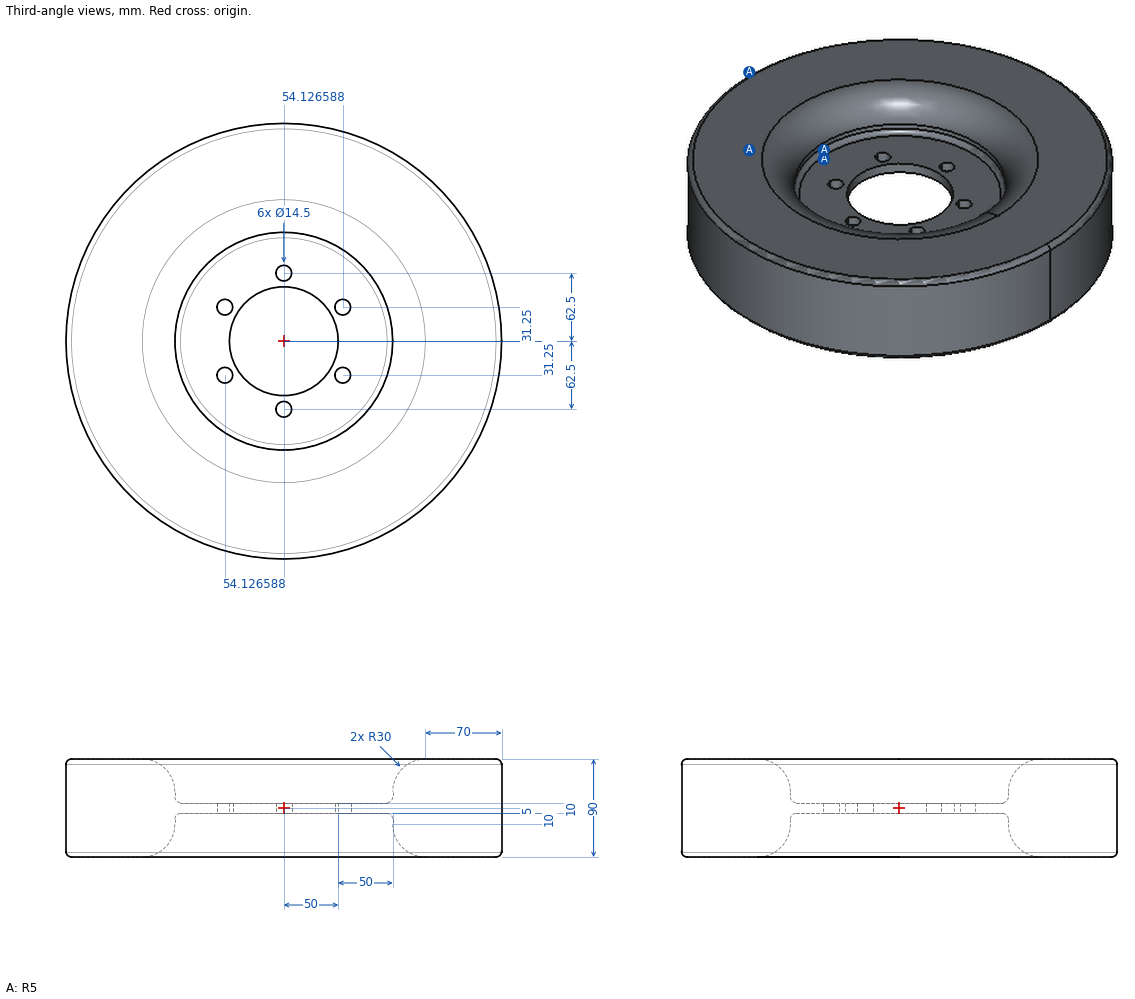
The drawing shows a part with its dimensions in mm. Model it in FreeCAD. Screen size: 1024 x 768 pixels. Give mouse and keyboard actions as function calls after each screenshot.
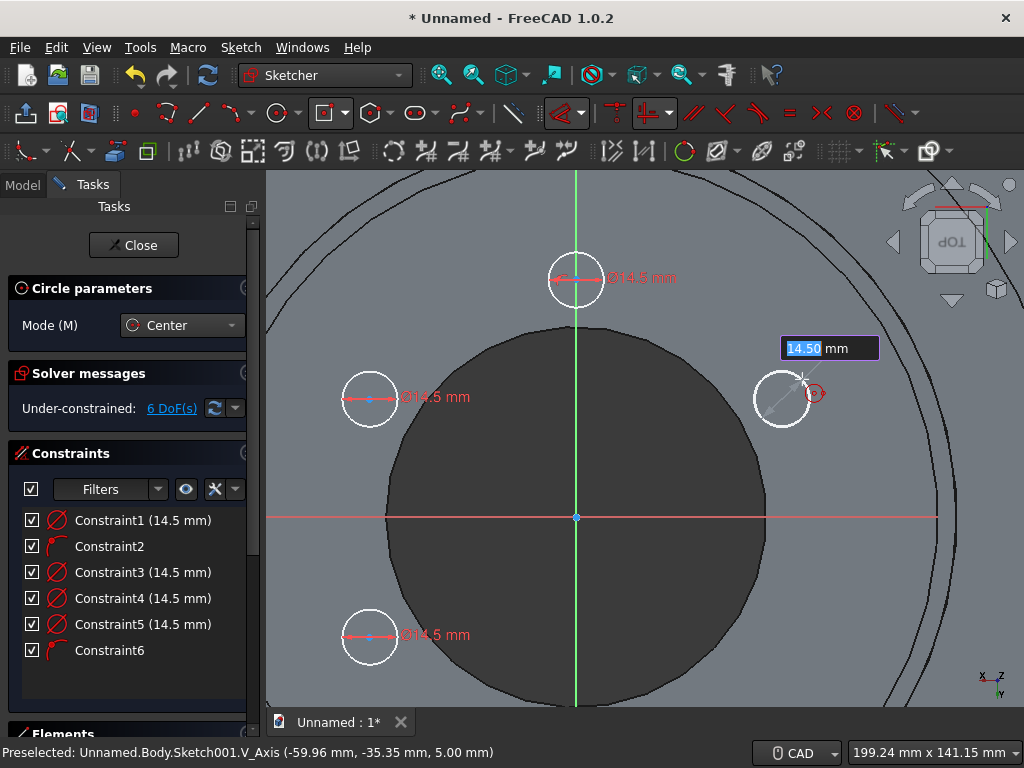
text(14.5)
key(Return)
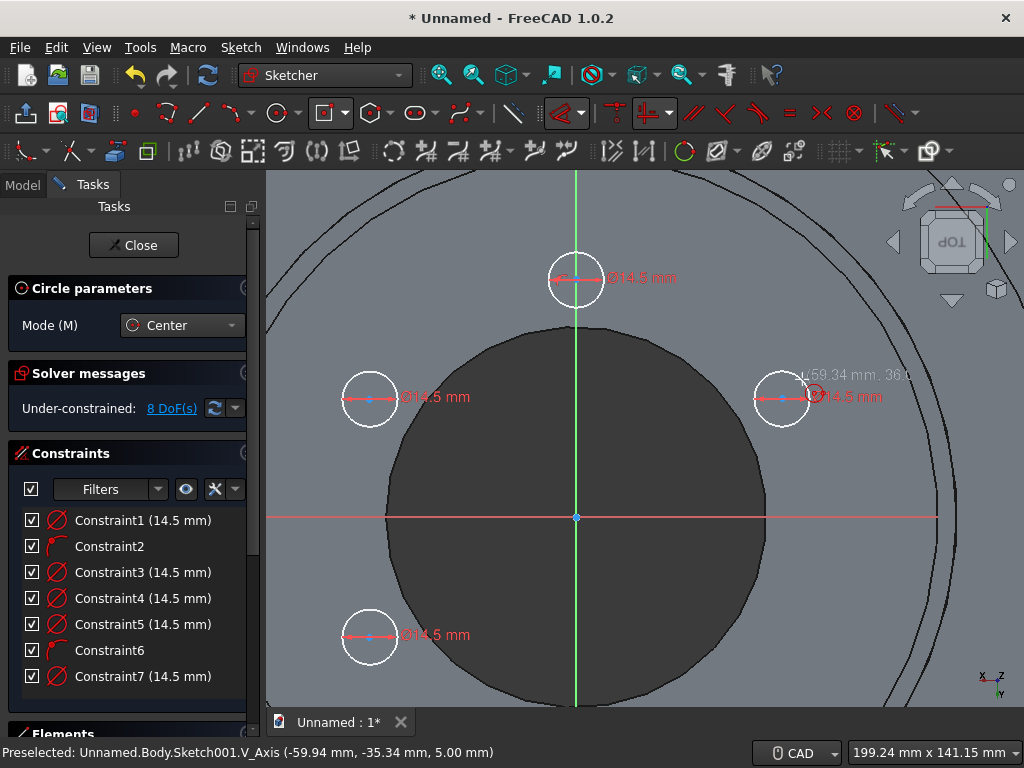
click(782, 636)
move(802, 617)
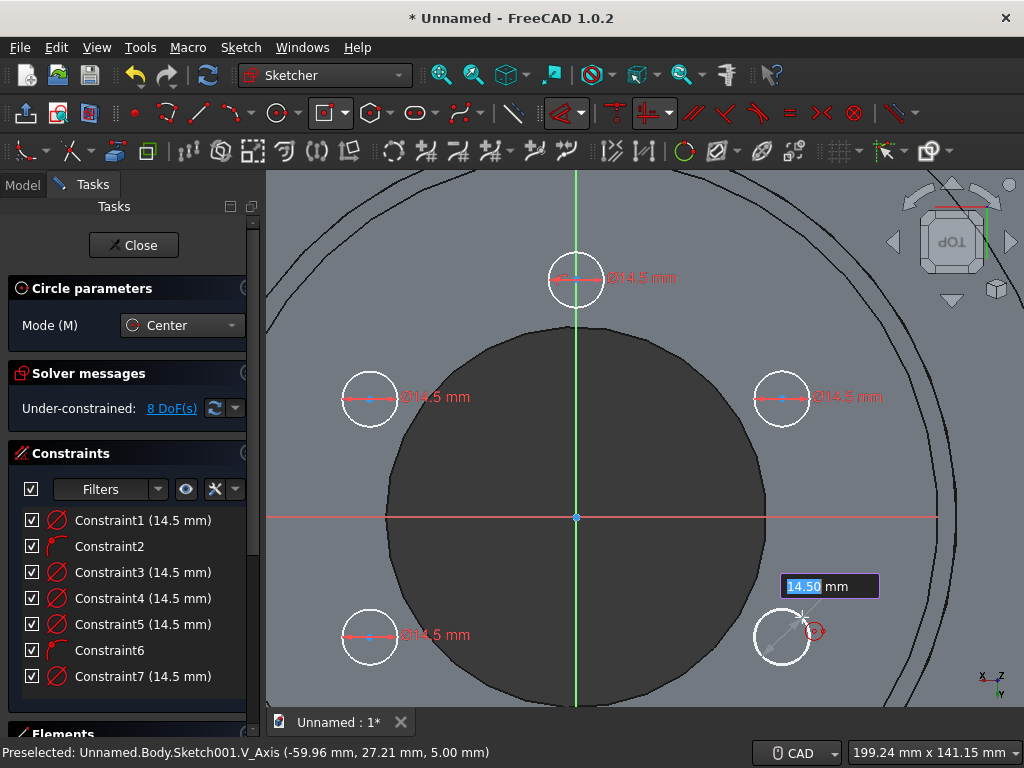
text(14.5)
key(Return)
key(Escape)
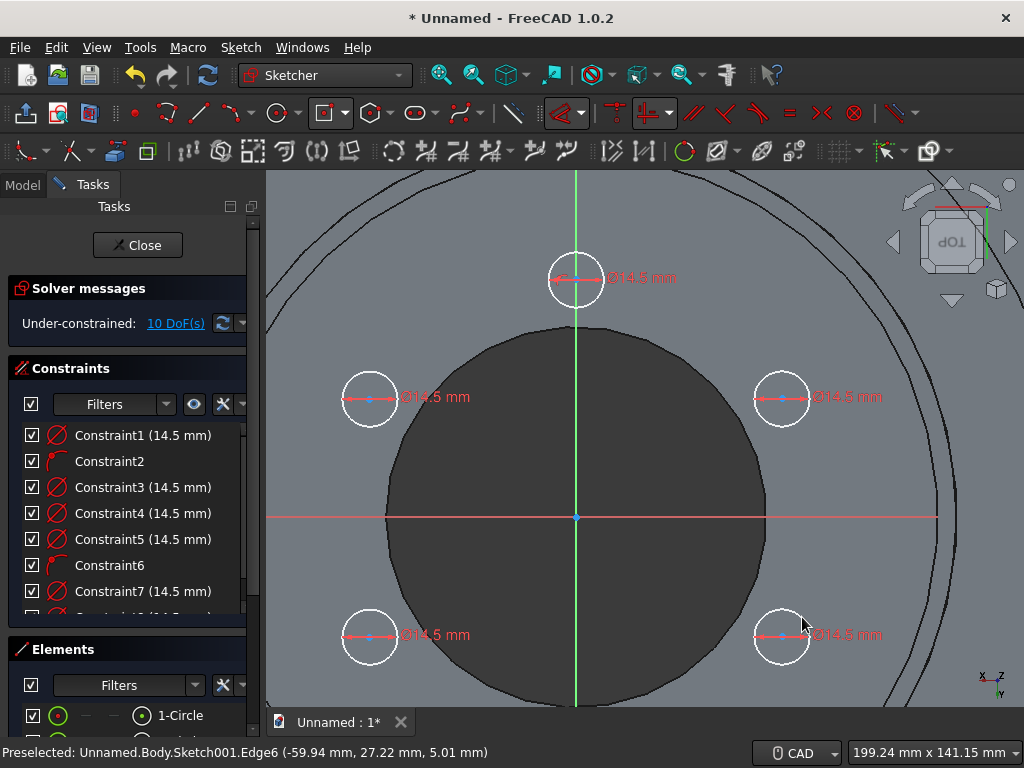
scroll(577, 278, down, 2)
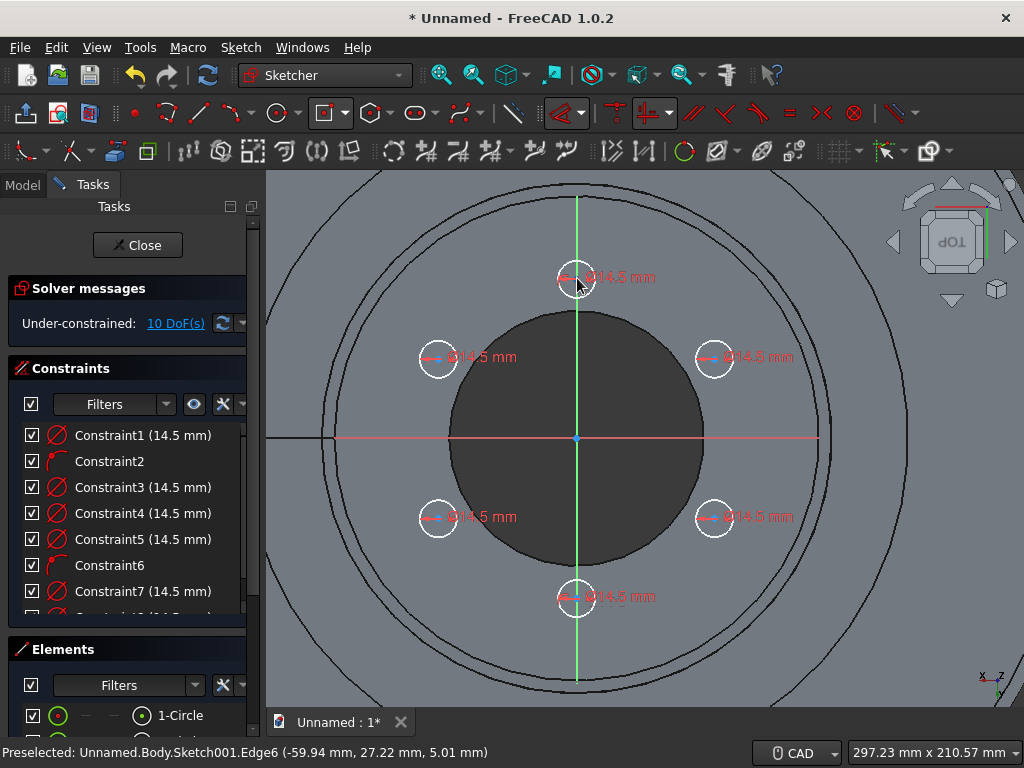
click(577, 599)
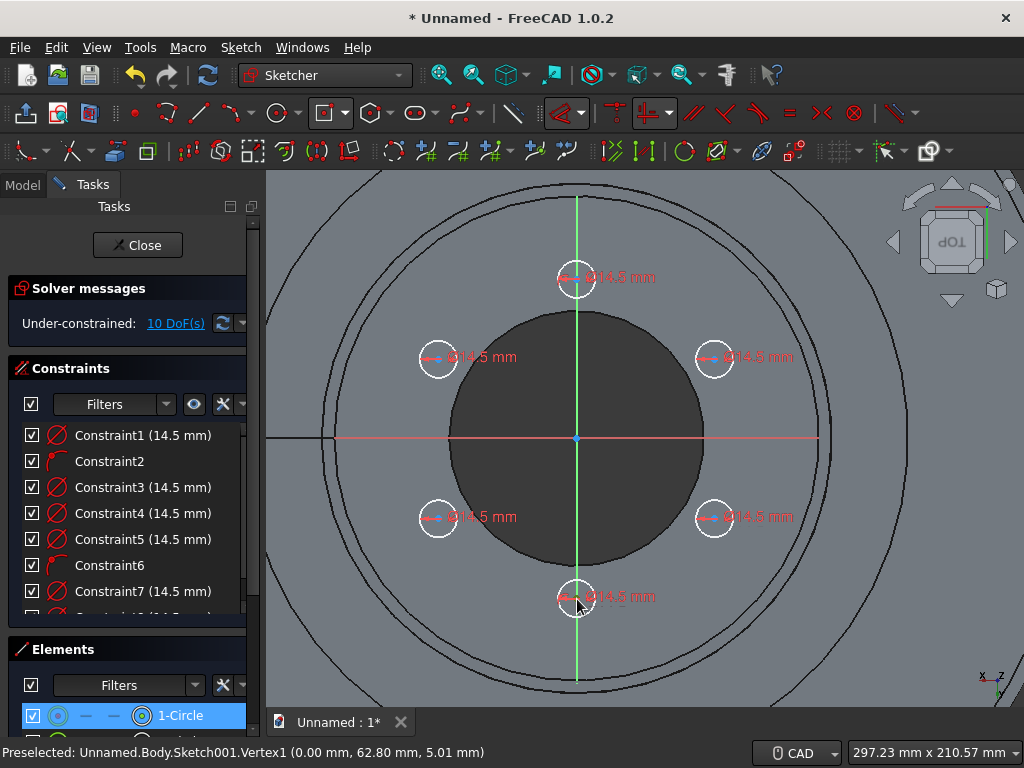
click(584, 114)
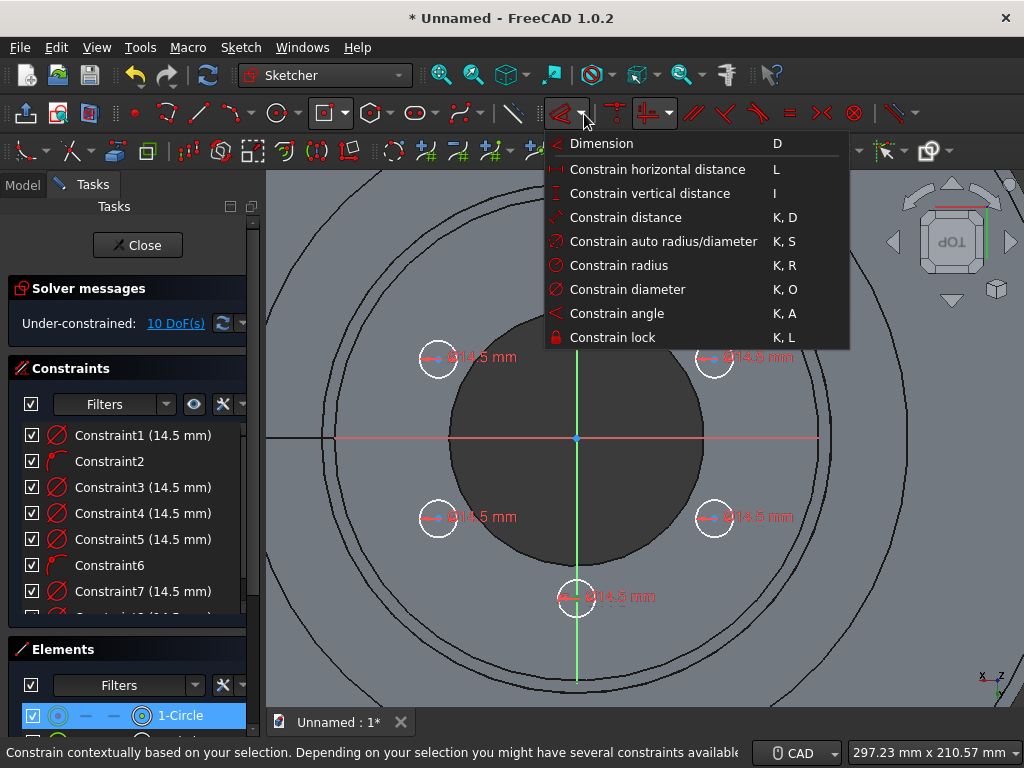
click(697, 193)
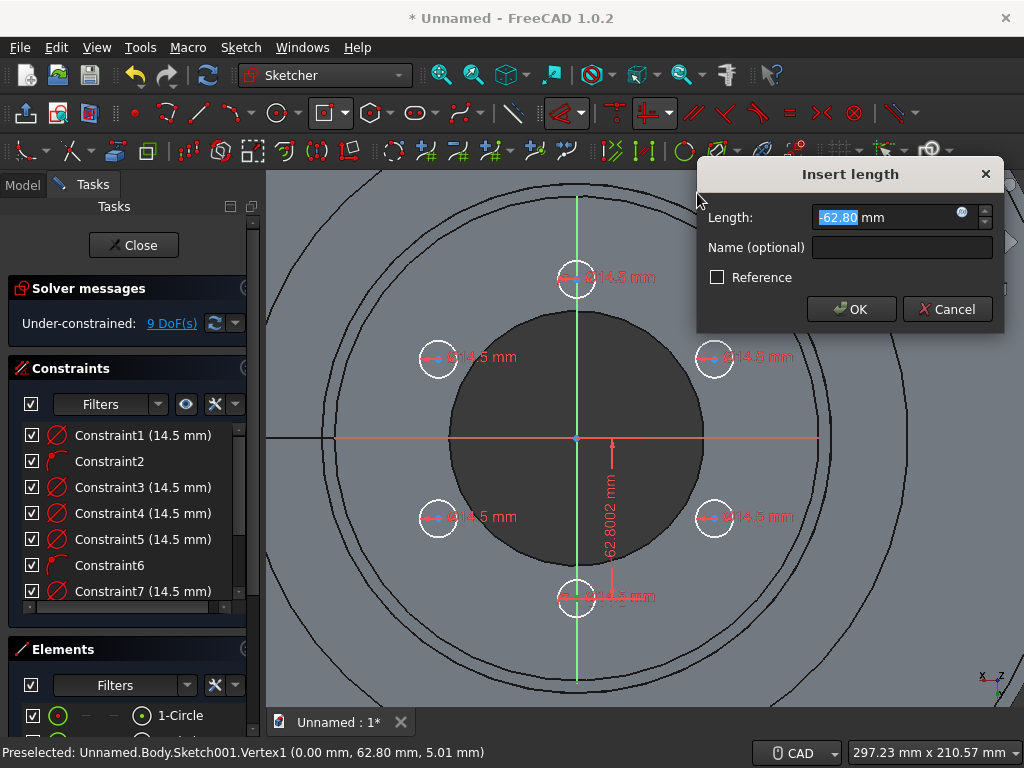
text(-62.5)
key(Return)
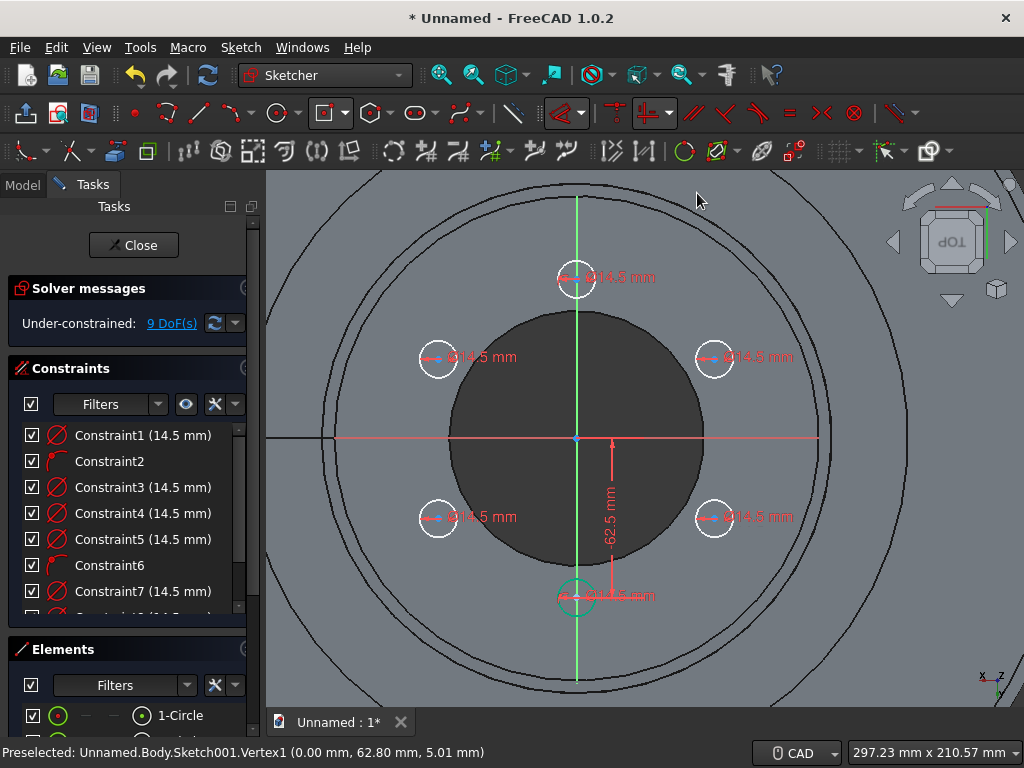
click(577, 279)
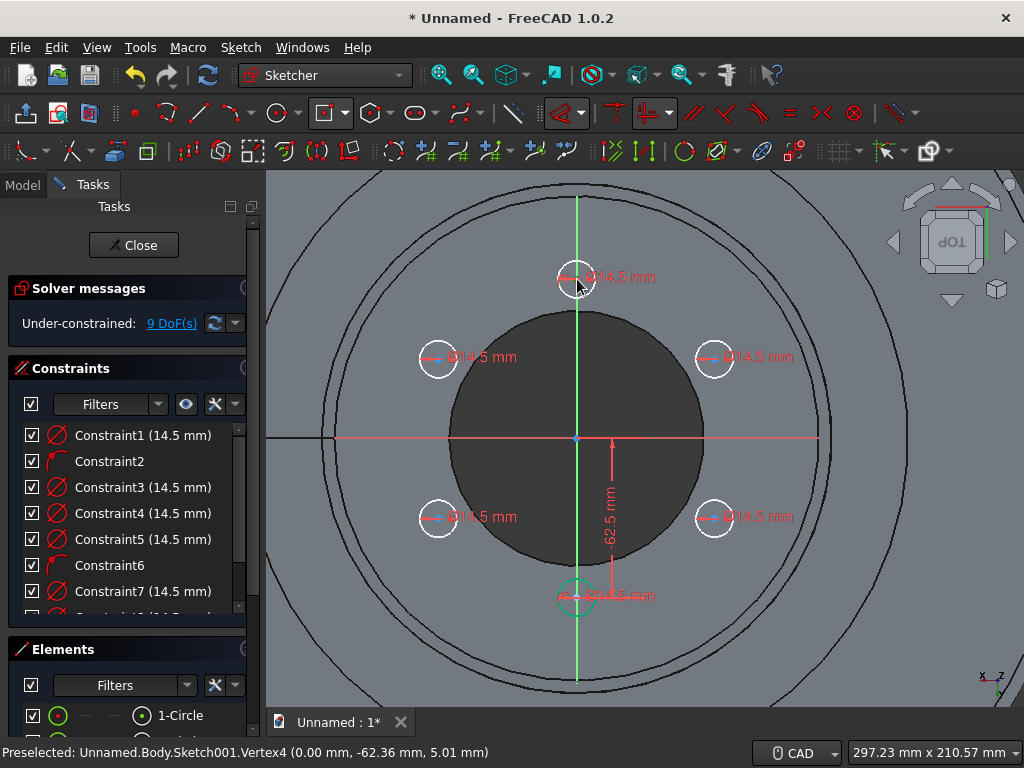
click(584, 114)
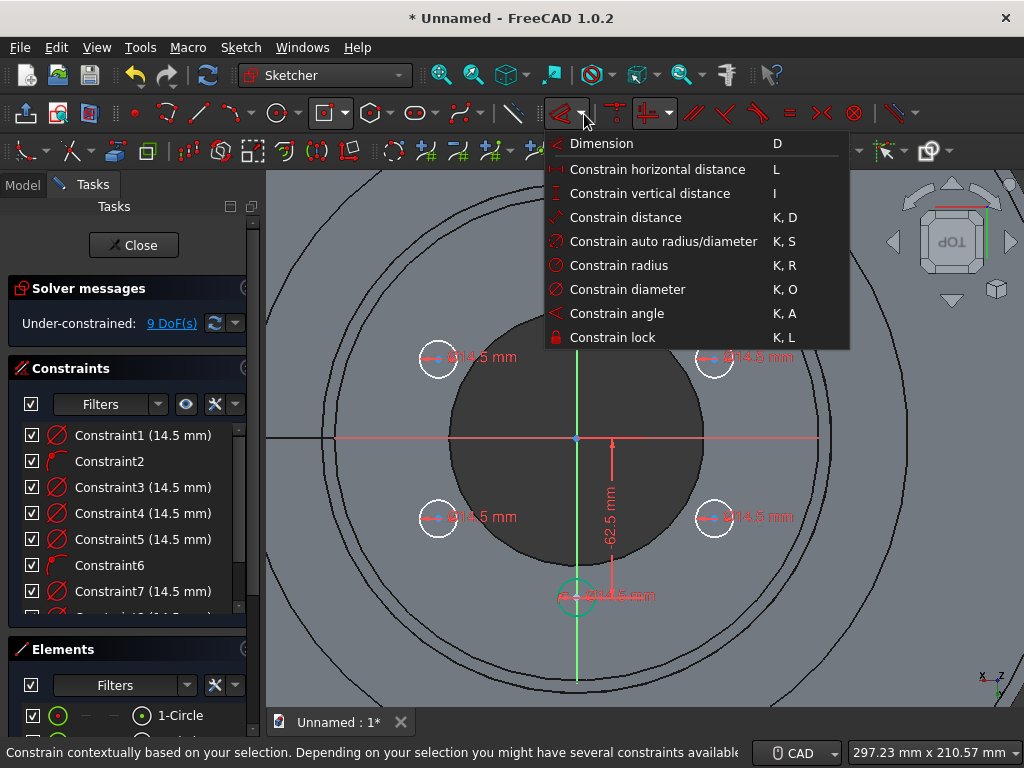
click(697, 193)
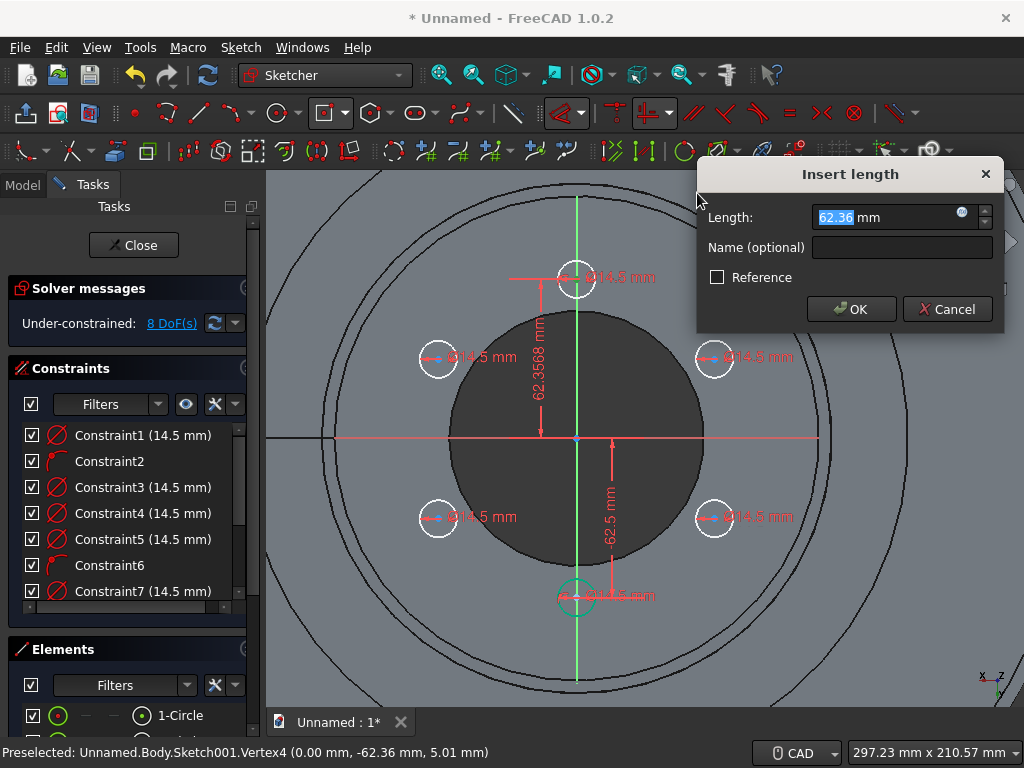
text(62.5)
key(Return)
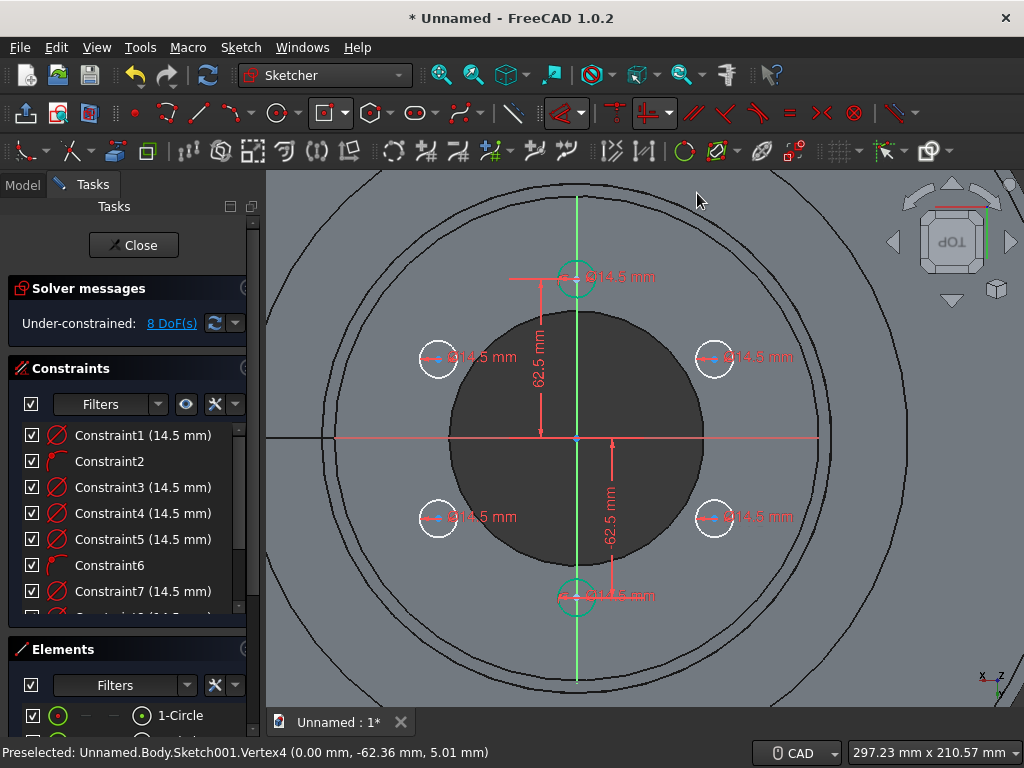
click(438, 519)